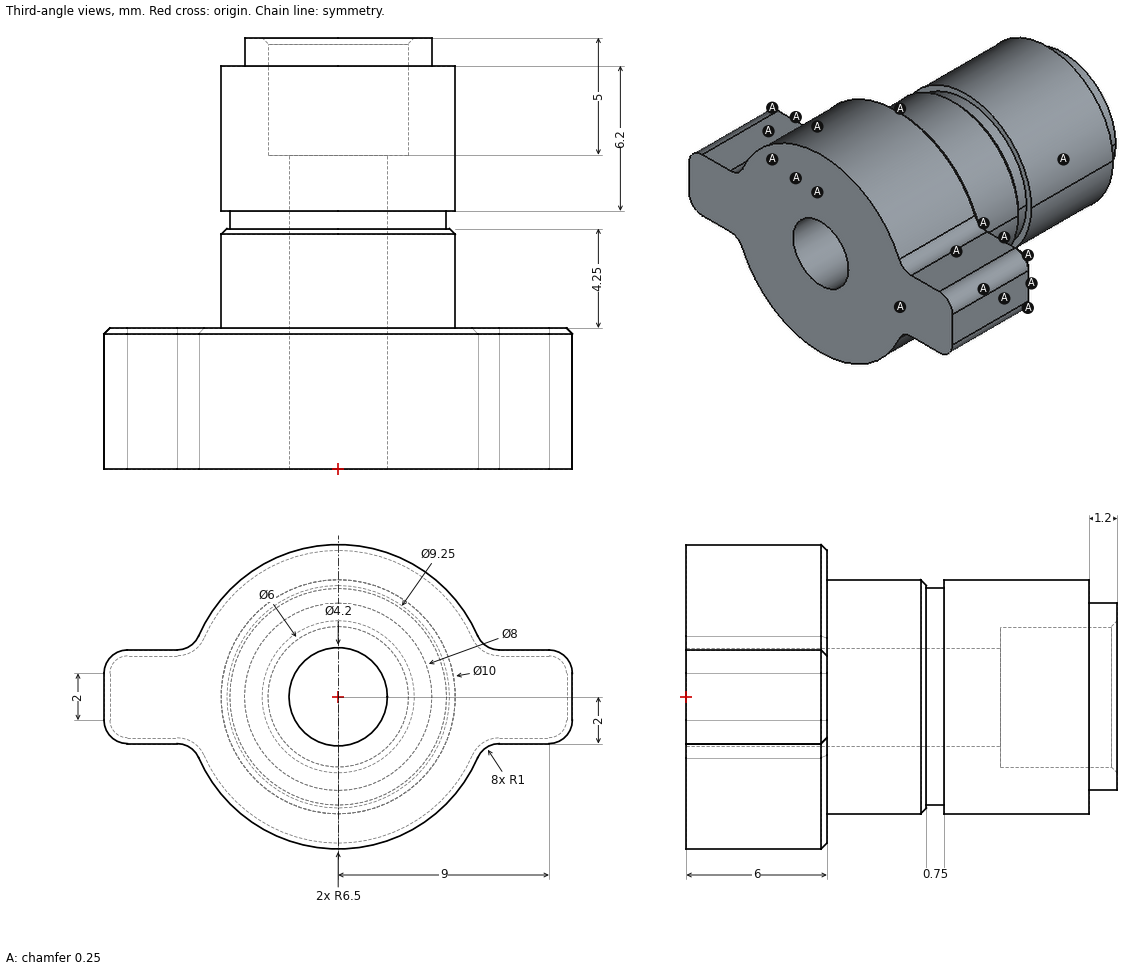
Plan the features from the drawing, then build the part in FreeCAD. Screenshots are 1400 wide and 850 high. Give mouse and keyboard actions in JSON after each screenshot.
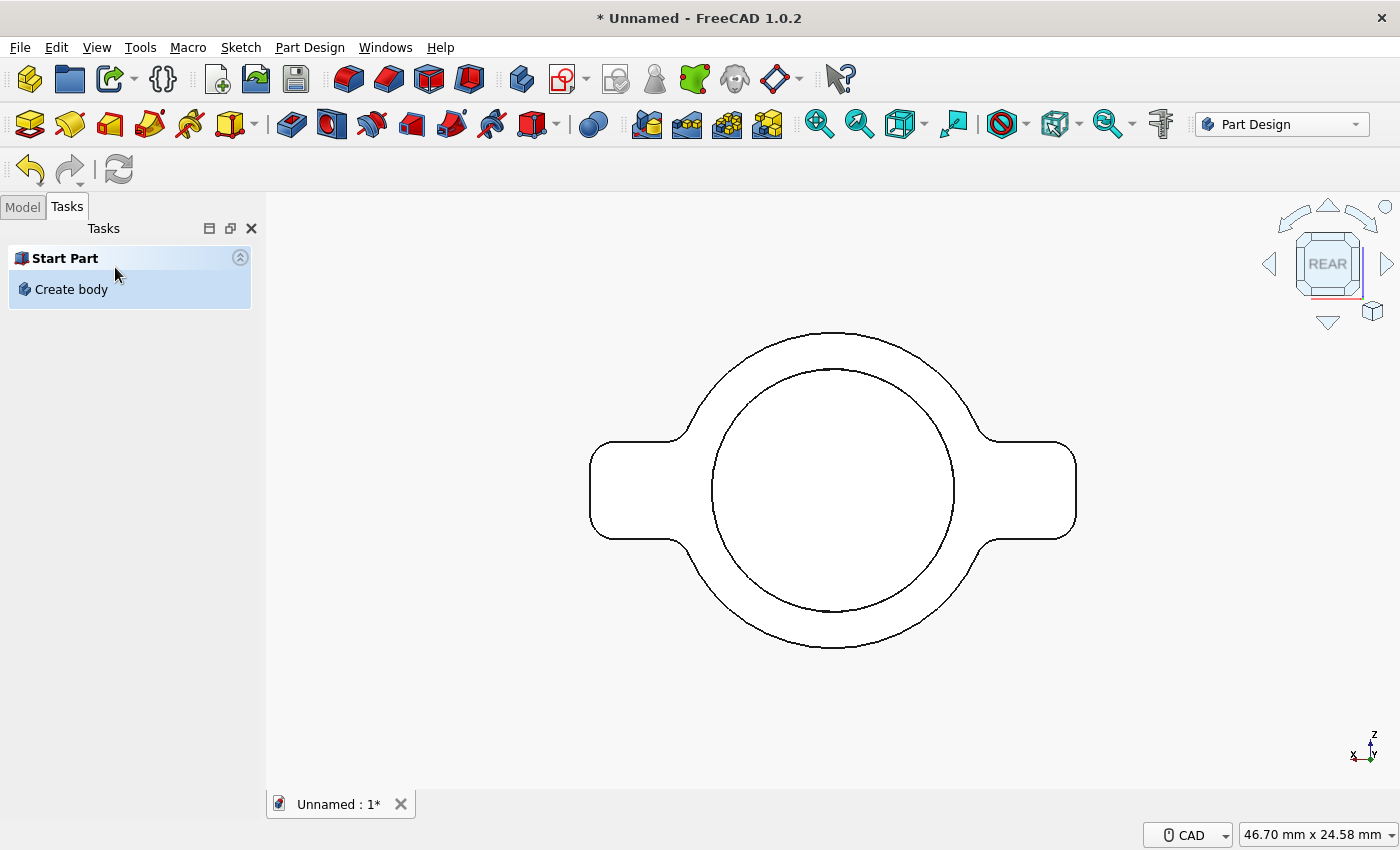
{"action": "left_click", "coordinate": [833, 490]}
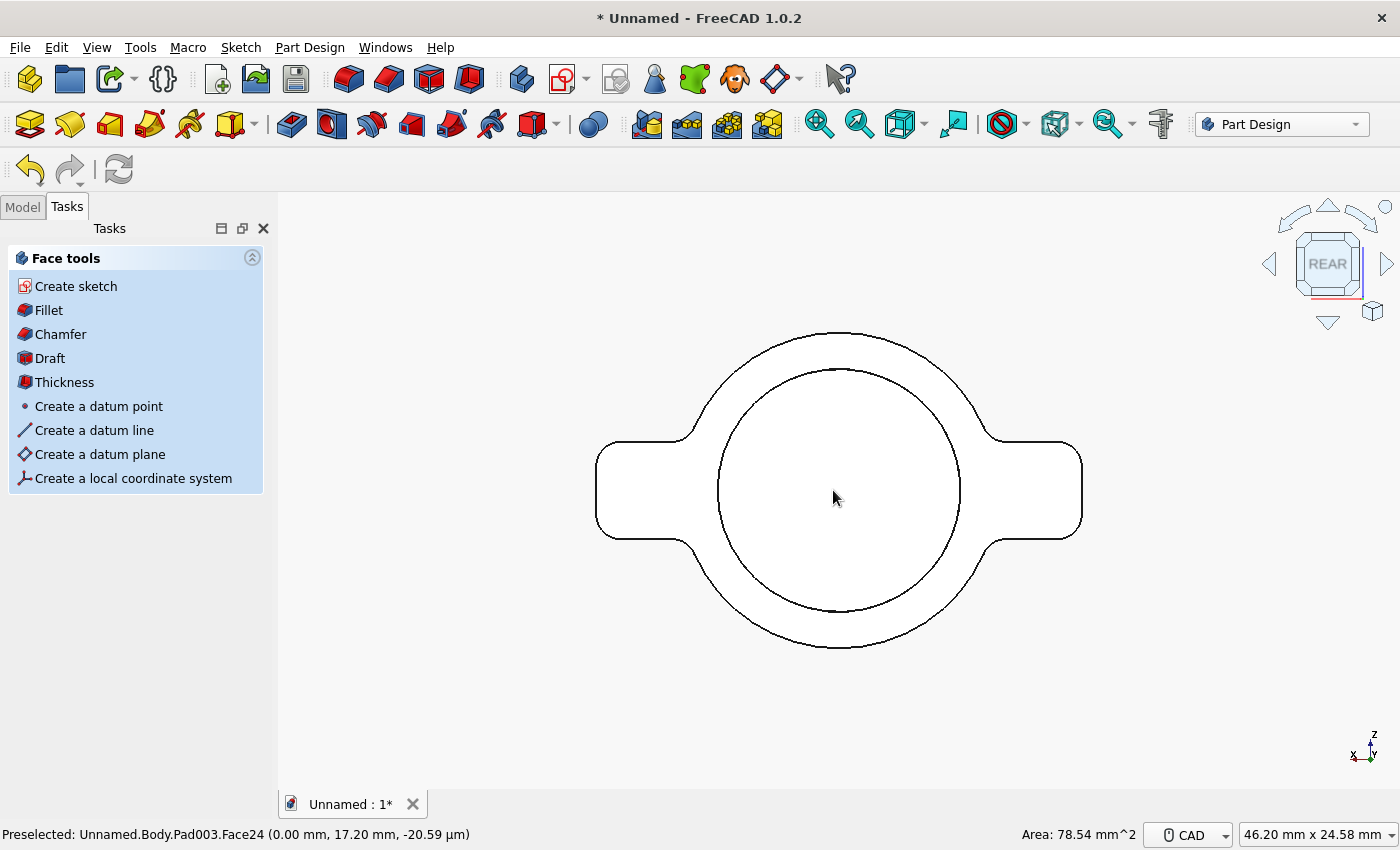
{"action": "left_click", "coordinate": [562, 80]}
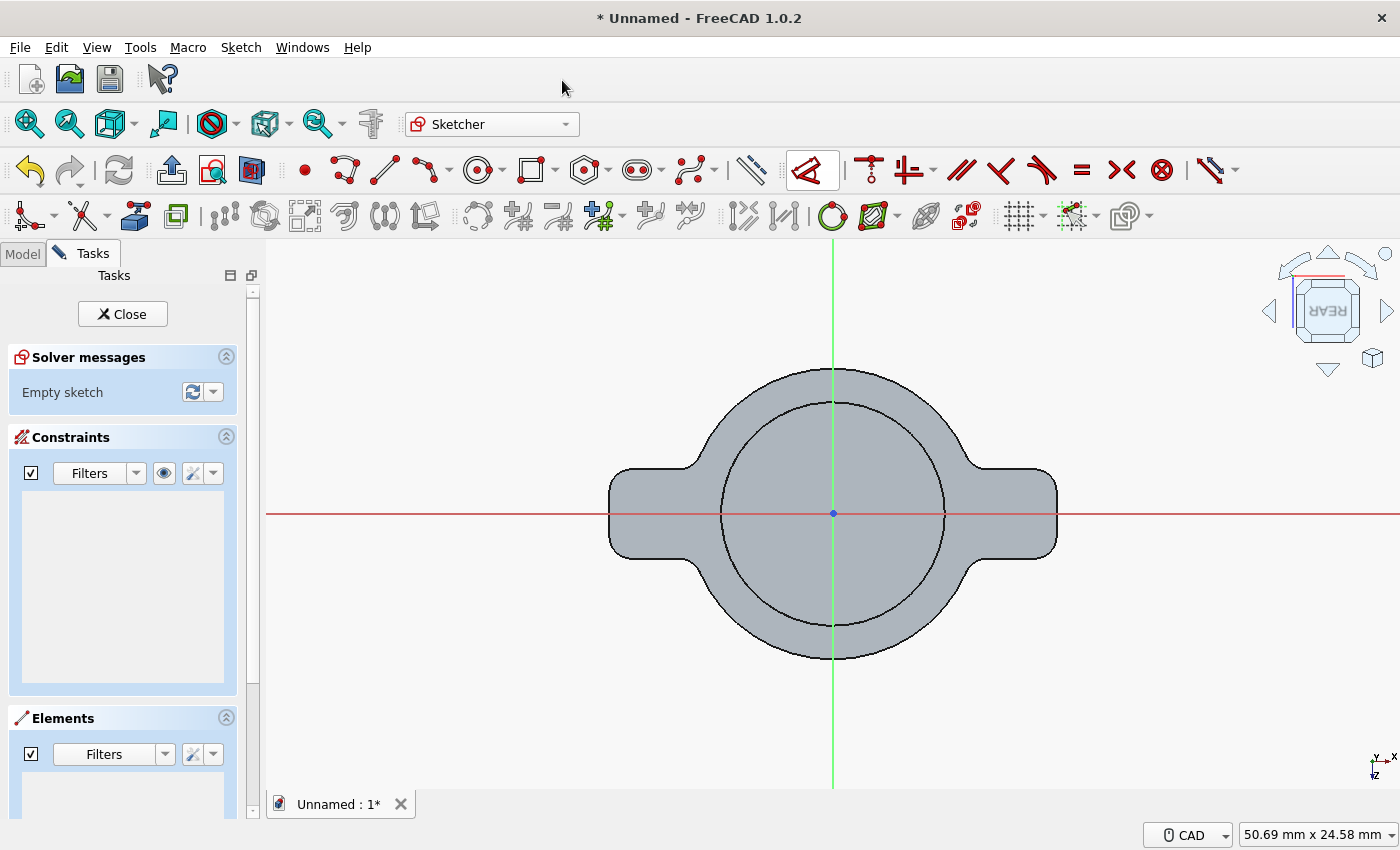
{"action": "scroll", "coordinate": [916, 514], "scroll_direction": "up", "scroll_amount": 3}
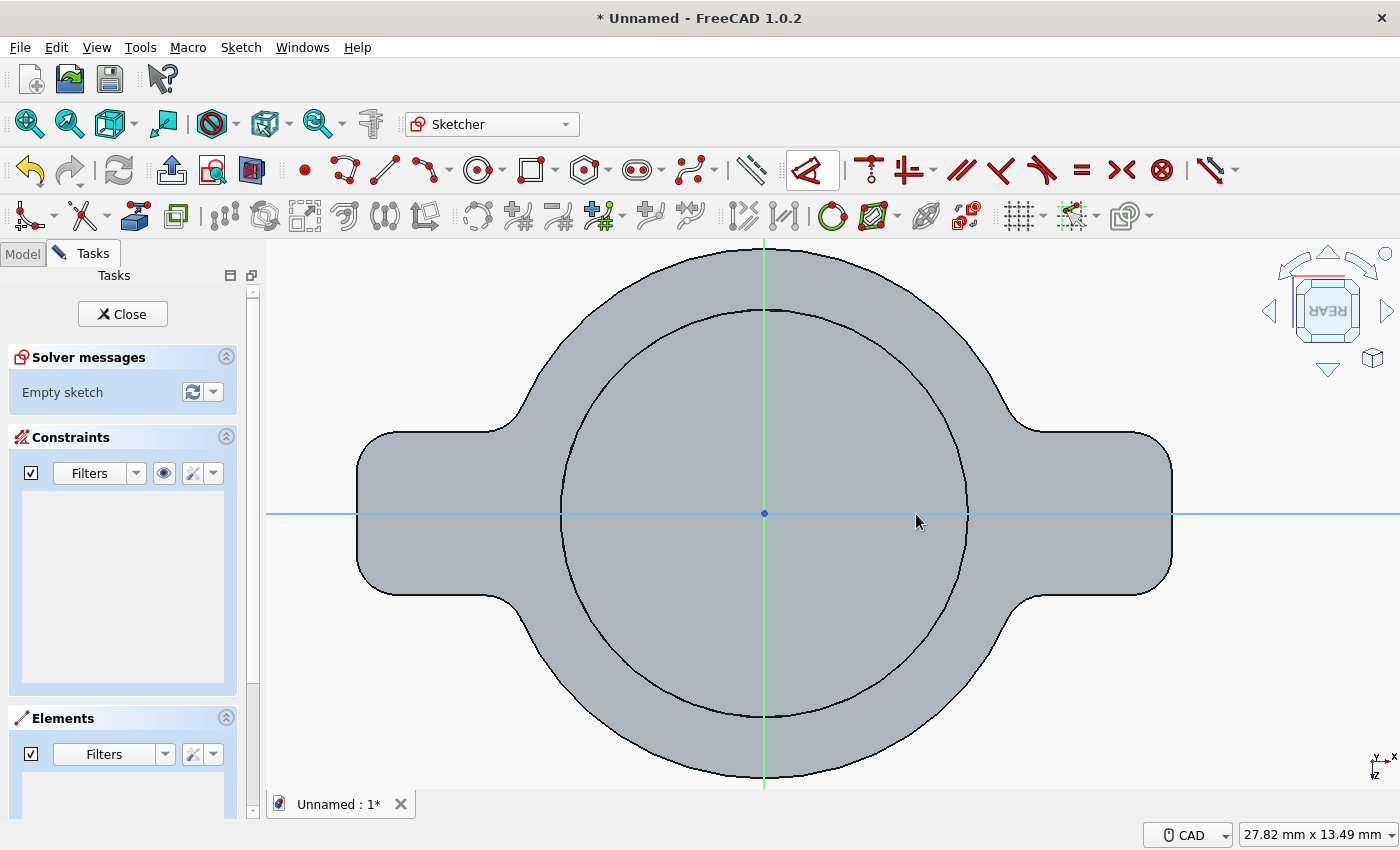
{"action": "left_click", "coordinate": [478, 170]}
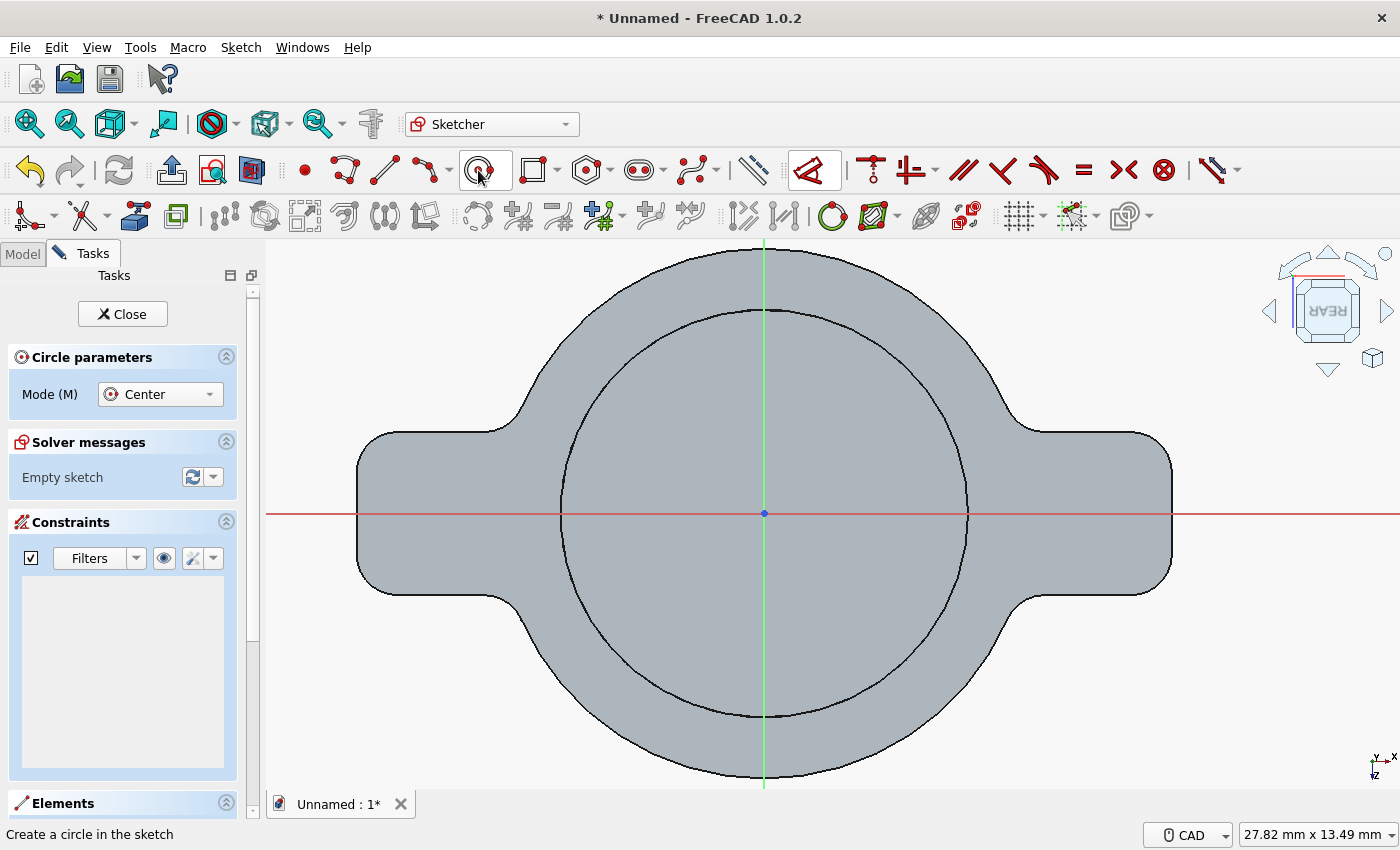
{"action": "left_click", "coordinate": [764, 514]}
{"action": "mouse_move", "coordinate": [880, 398]}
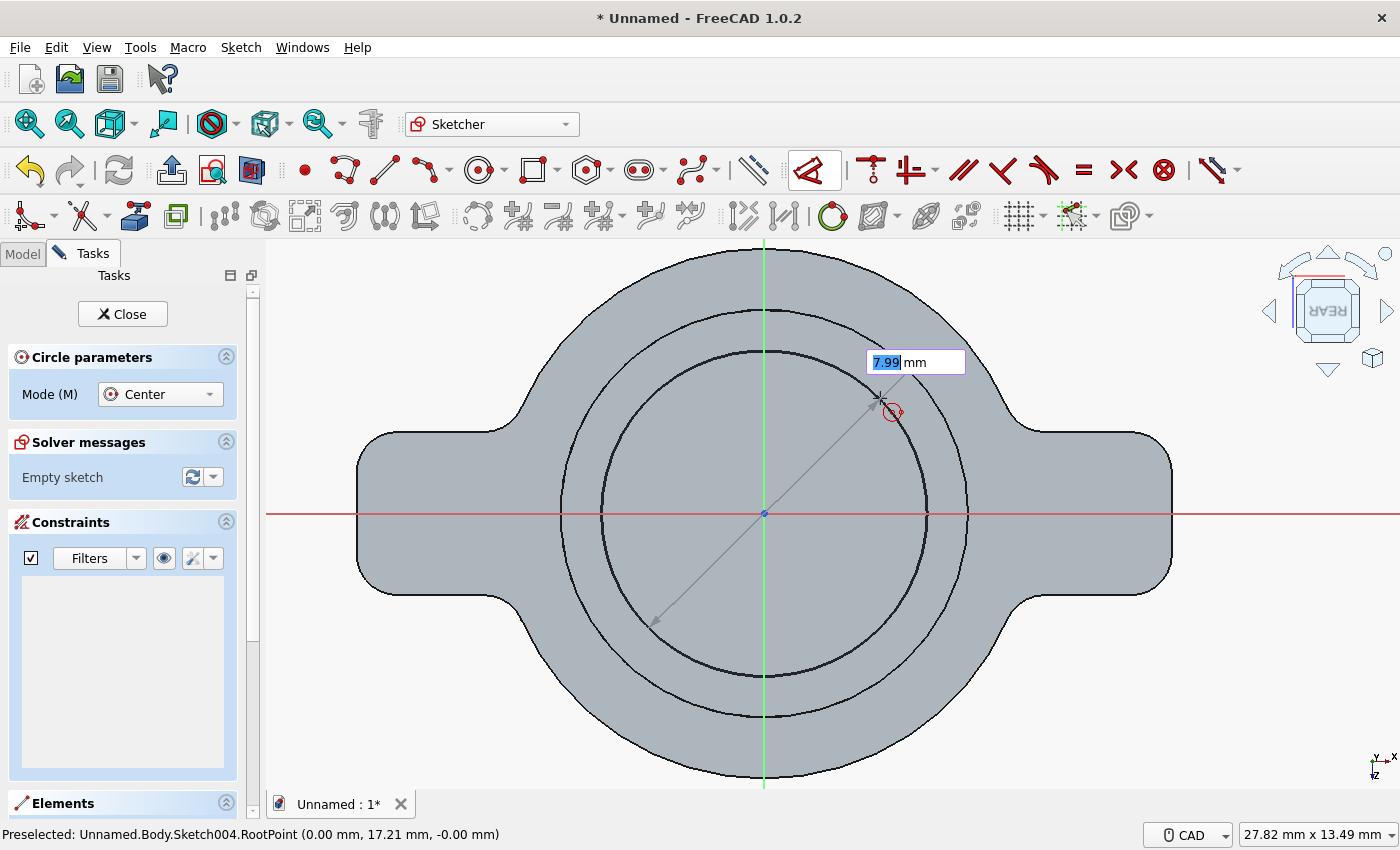
{"action": "type", "text": "8"}
{"action": "key", "text": "Return"}
{"action": "key", "text": "Escape"}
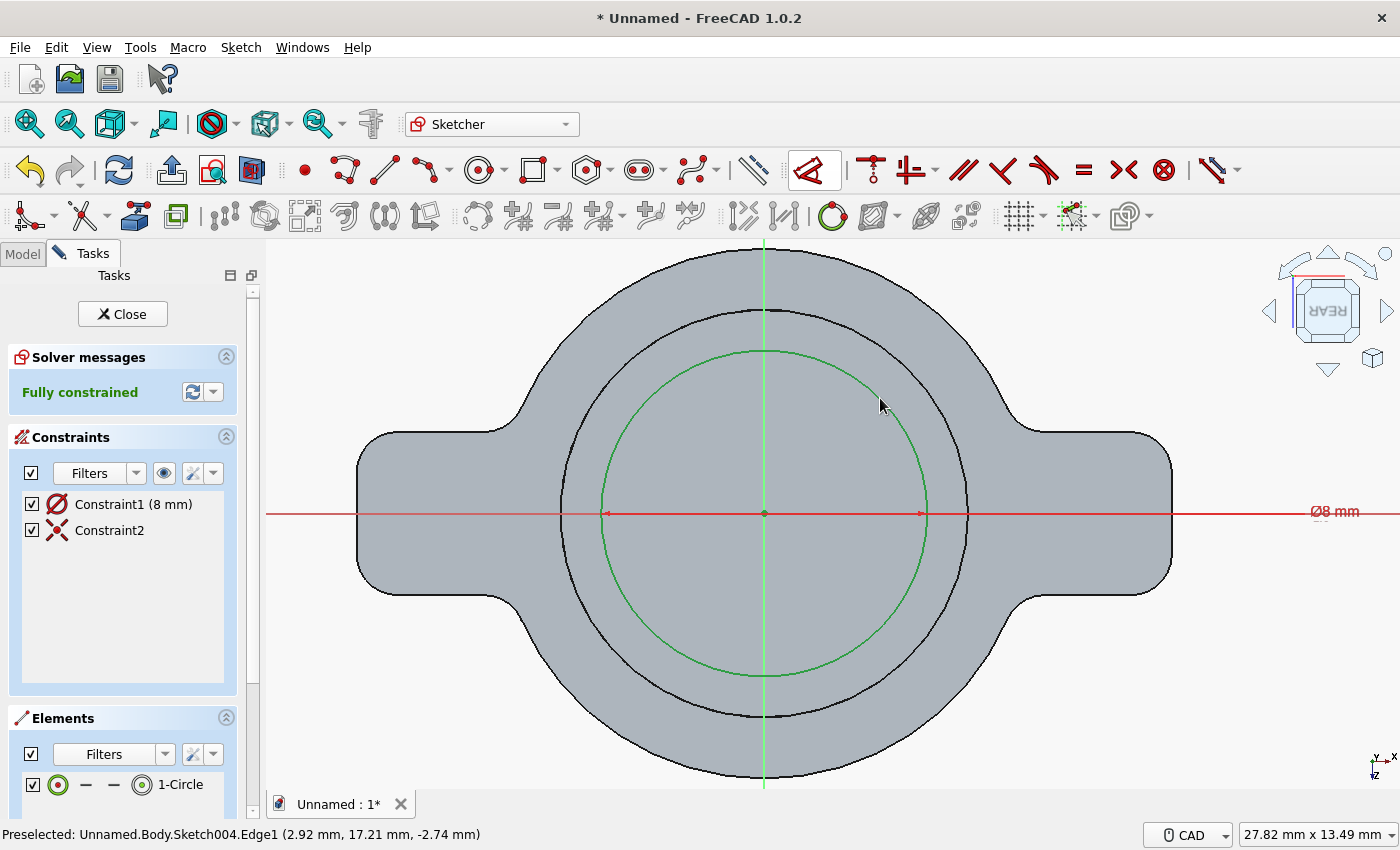
{"action": "left_click", "coordinate": [123, 314]}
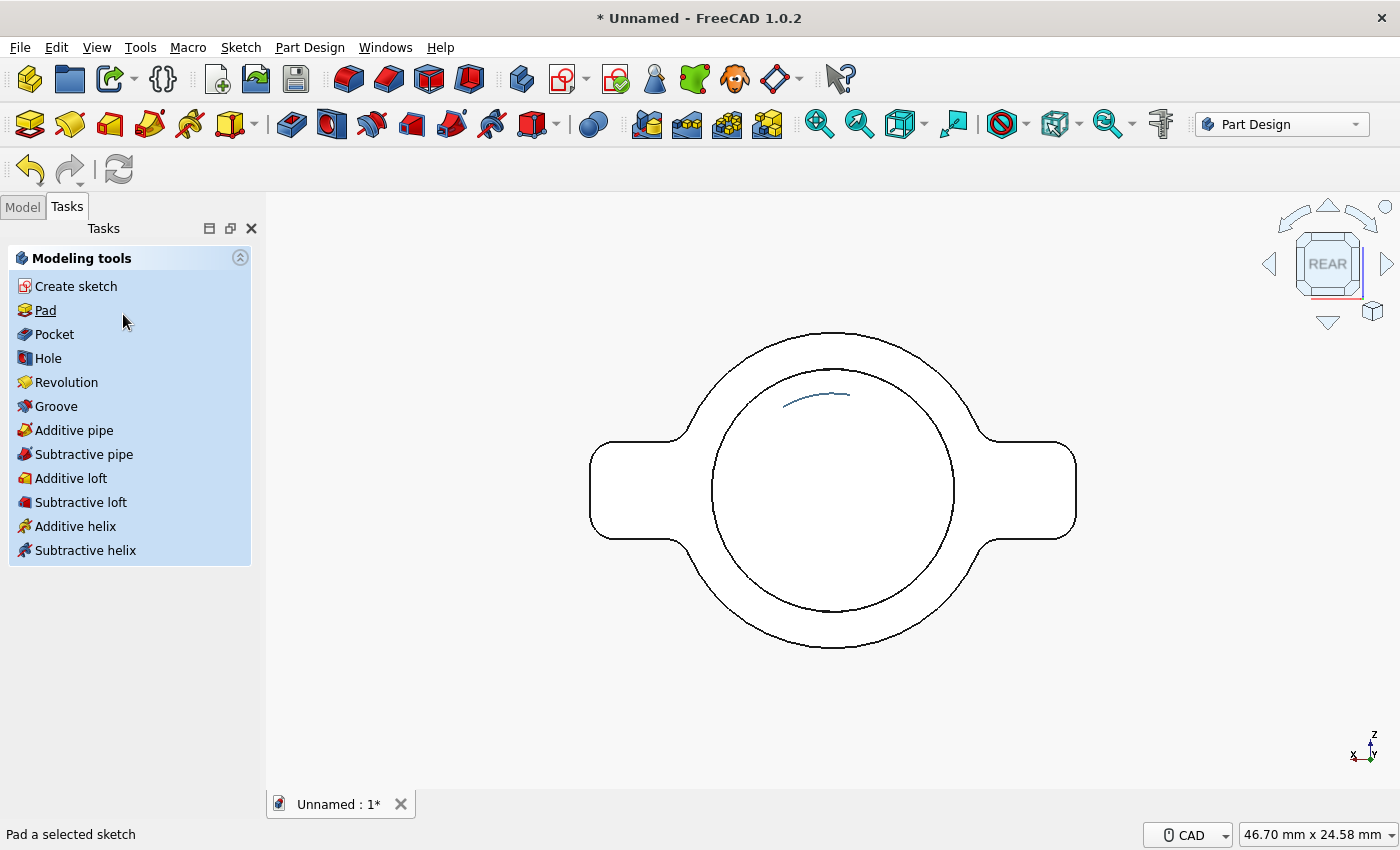
{"action": "left_click", "coordinate": [30, 124]}